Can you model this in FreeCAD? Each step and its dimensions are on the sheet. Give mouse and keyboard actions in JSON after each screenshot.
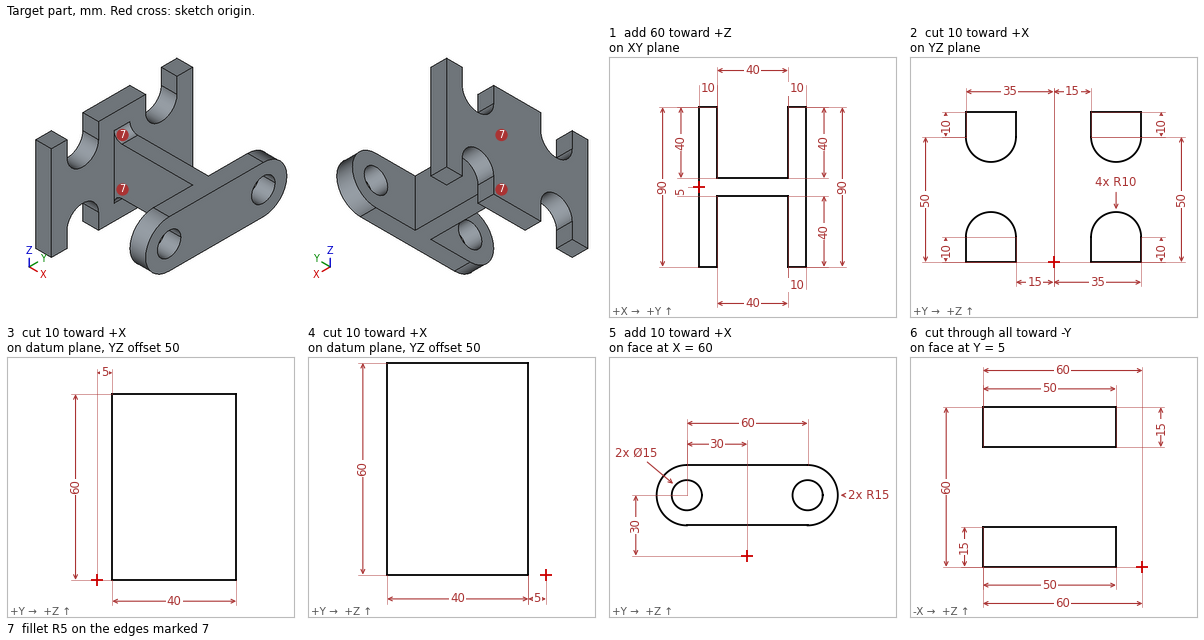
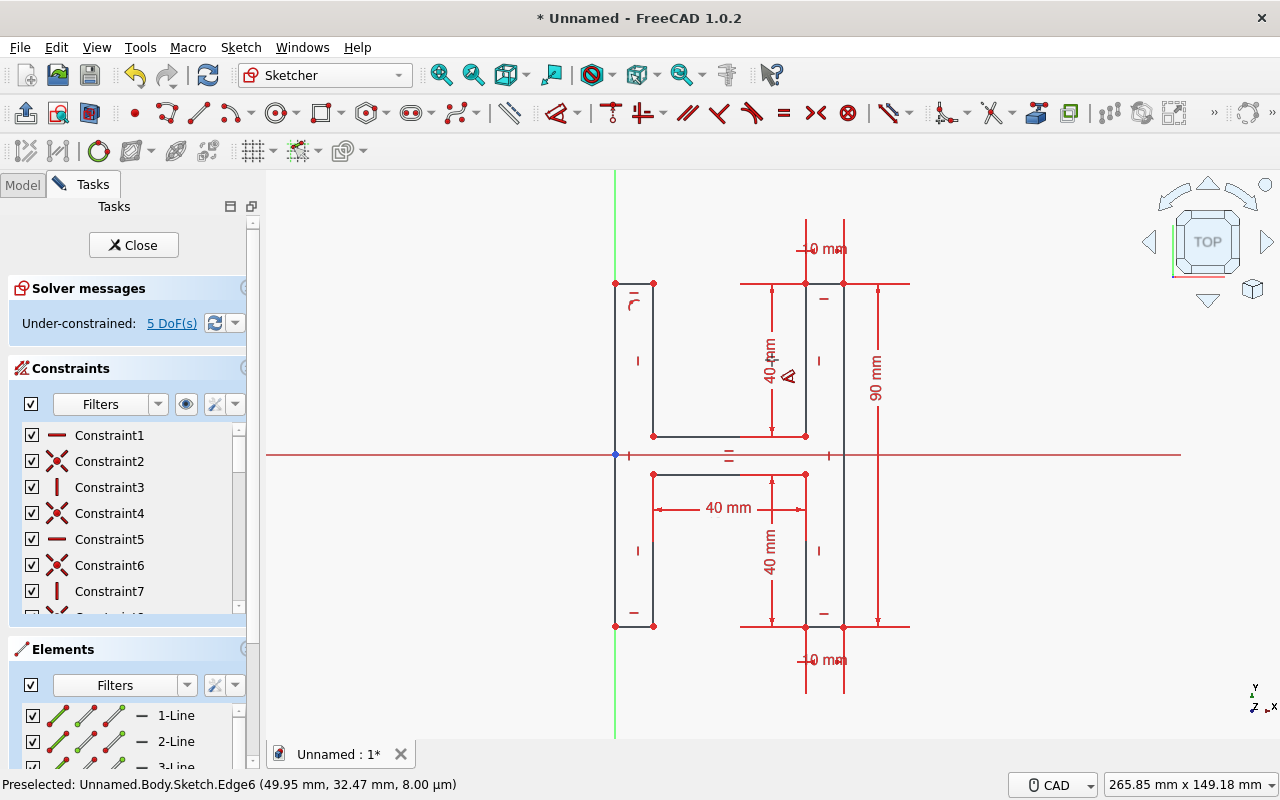
{"action": "left_click", "coordinate": [760, 437]}
{"action": "left_click", "coordinate": [729, 403]}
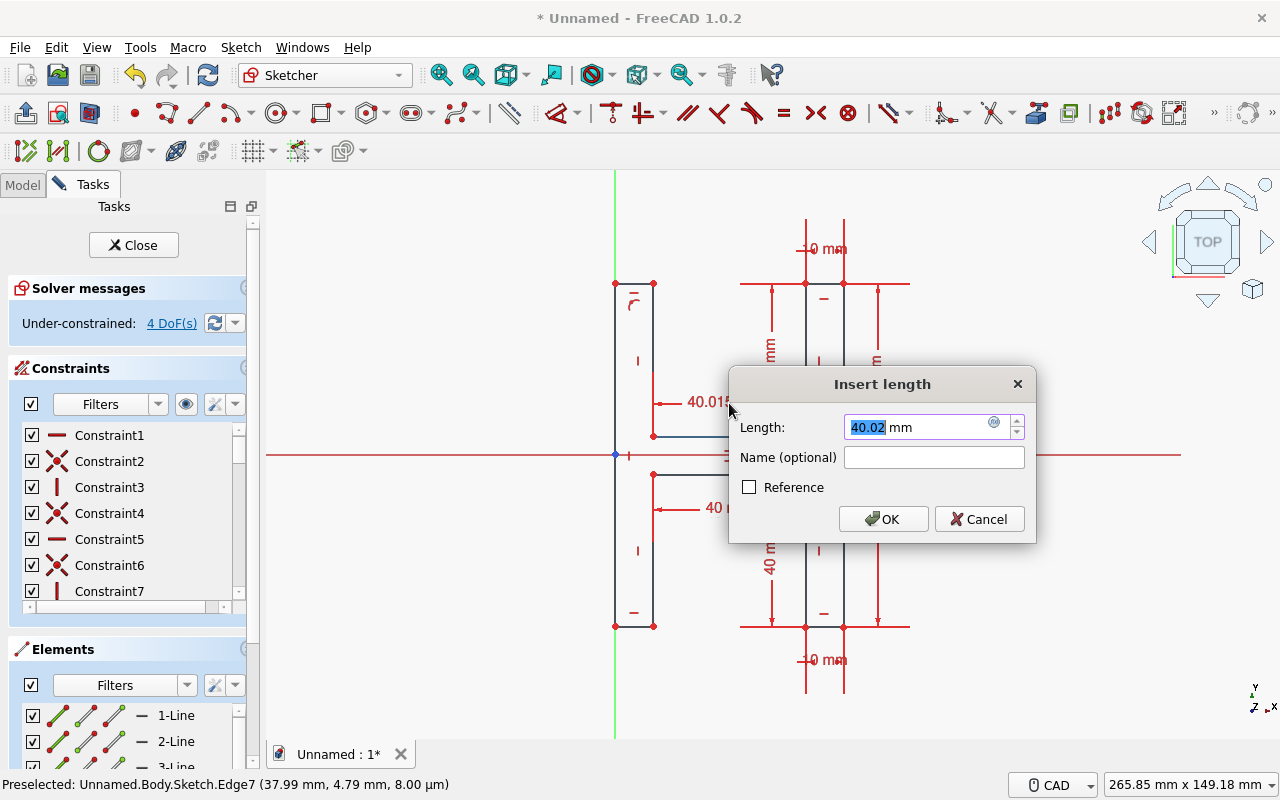
{"action": "type", "text": "40"}
{"action": "key", "text": "Return"}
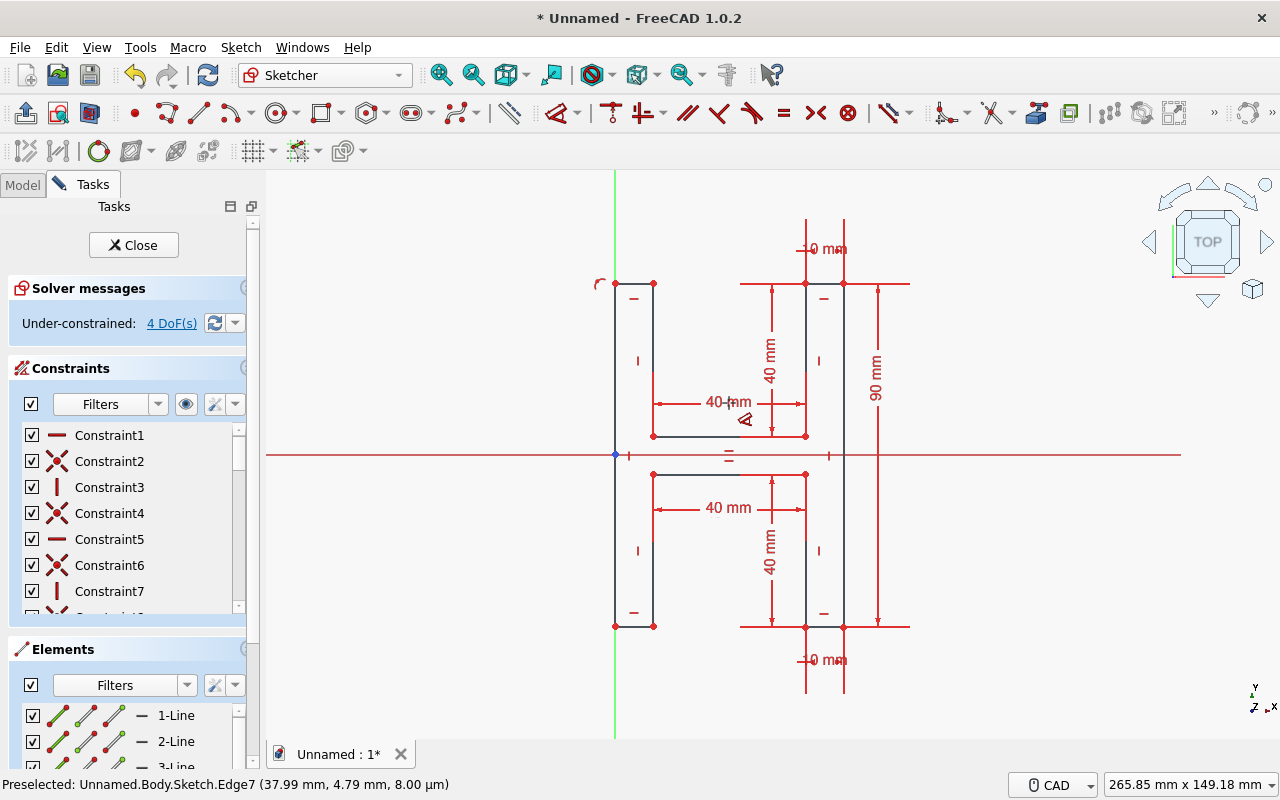
{"action": "left_click", "coordinate": [653, 391]}
{"action": "left_click", "coordinate": [687, 360]}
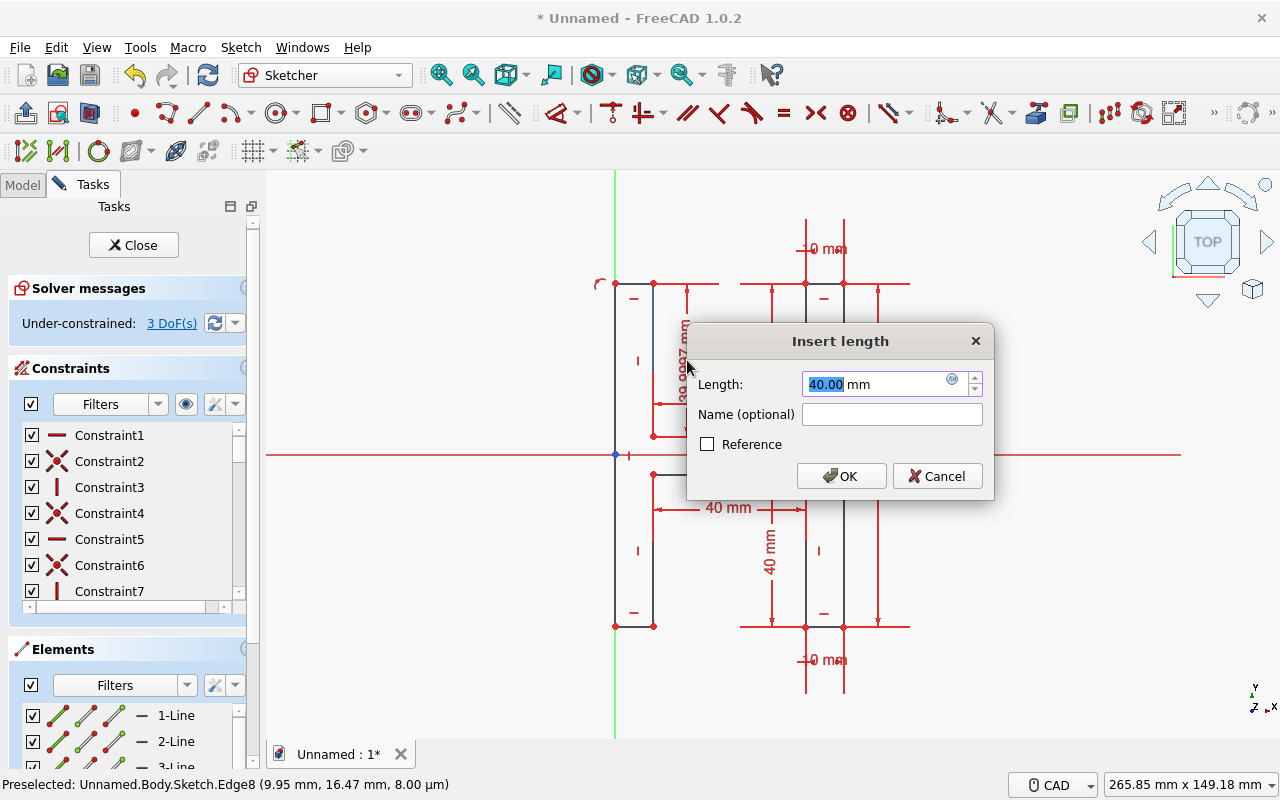
{"action": "type", "text": "40"}
{"action": "key", "text": "Return"}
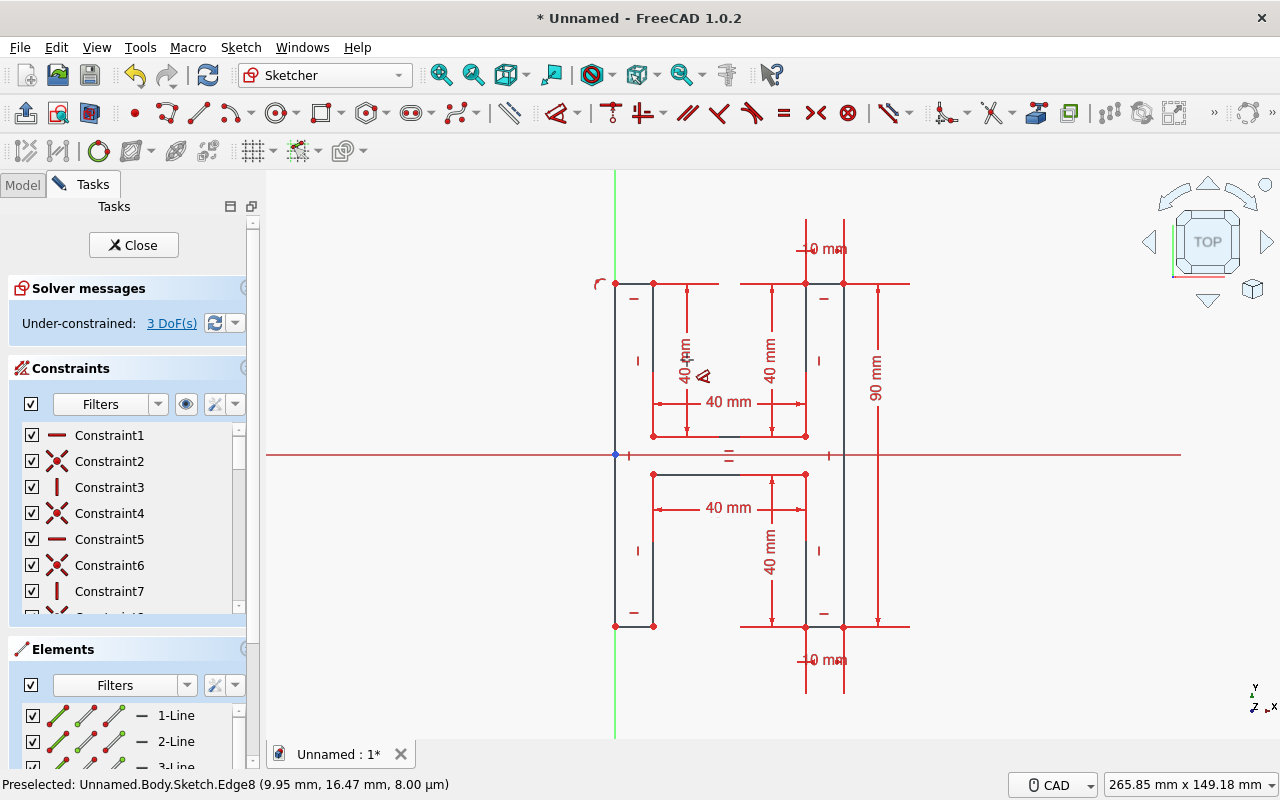
{"action": "left_click", "coordinate": [642, 284]}
{"action": "left_click", "coordinate": [634, 250]}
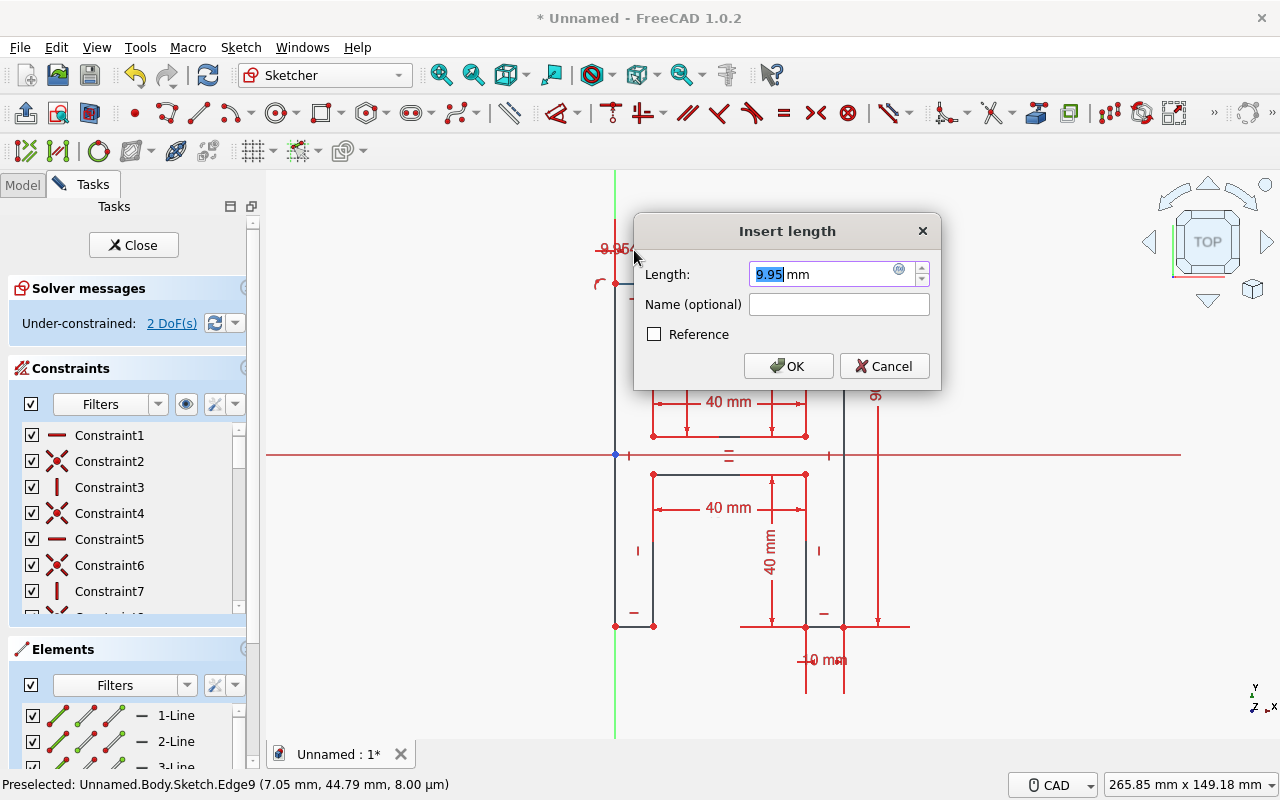
{"action": "type", "text": "10"}
{"action": "key", "text": "Return"}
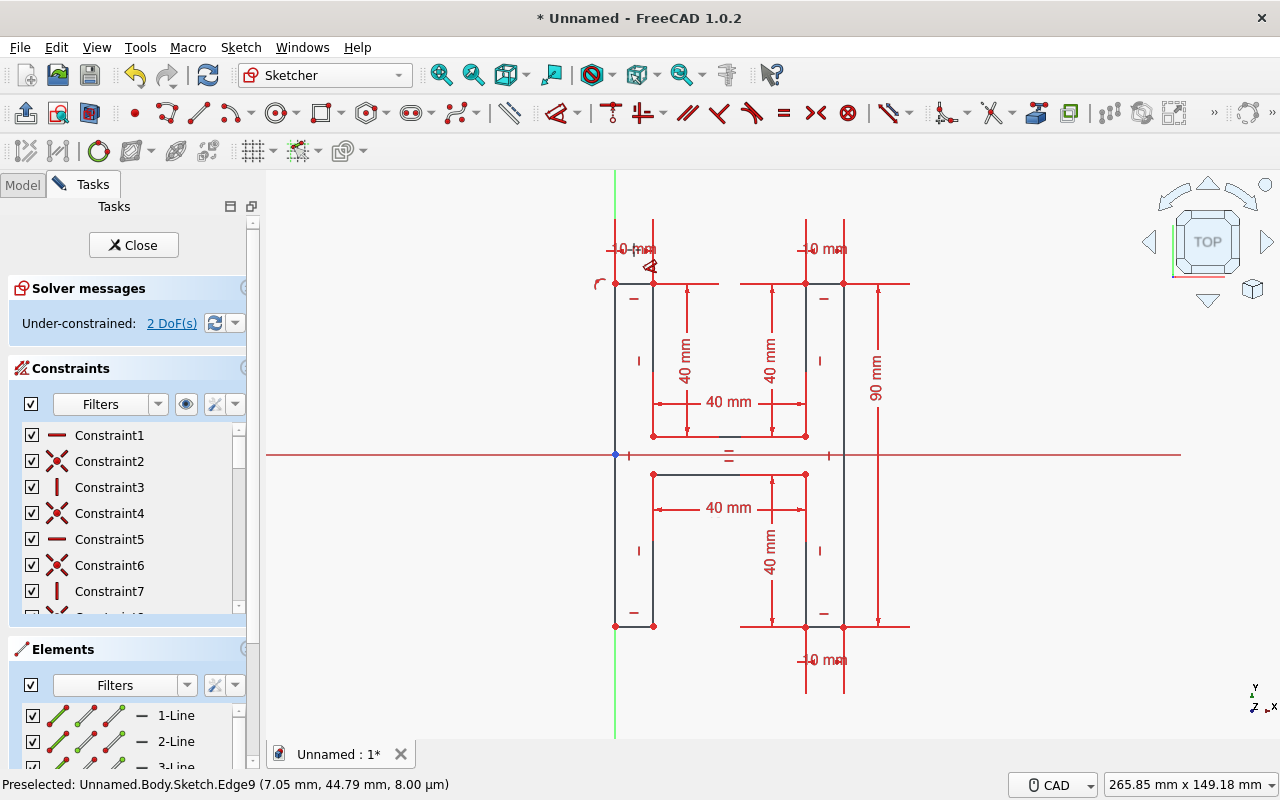
{"action": "left_click", "coordinate": [615, 387]}
{"action": "left_click", "coordinate": [581, 377]}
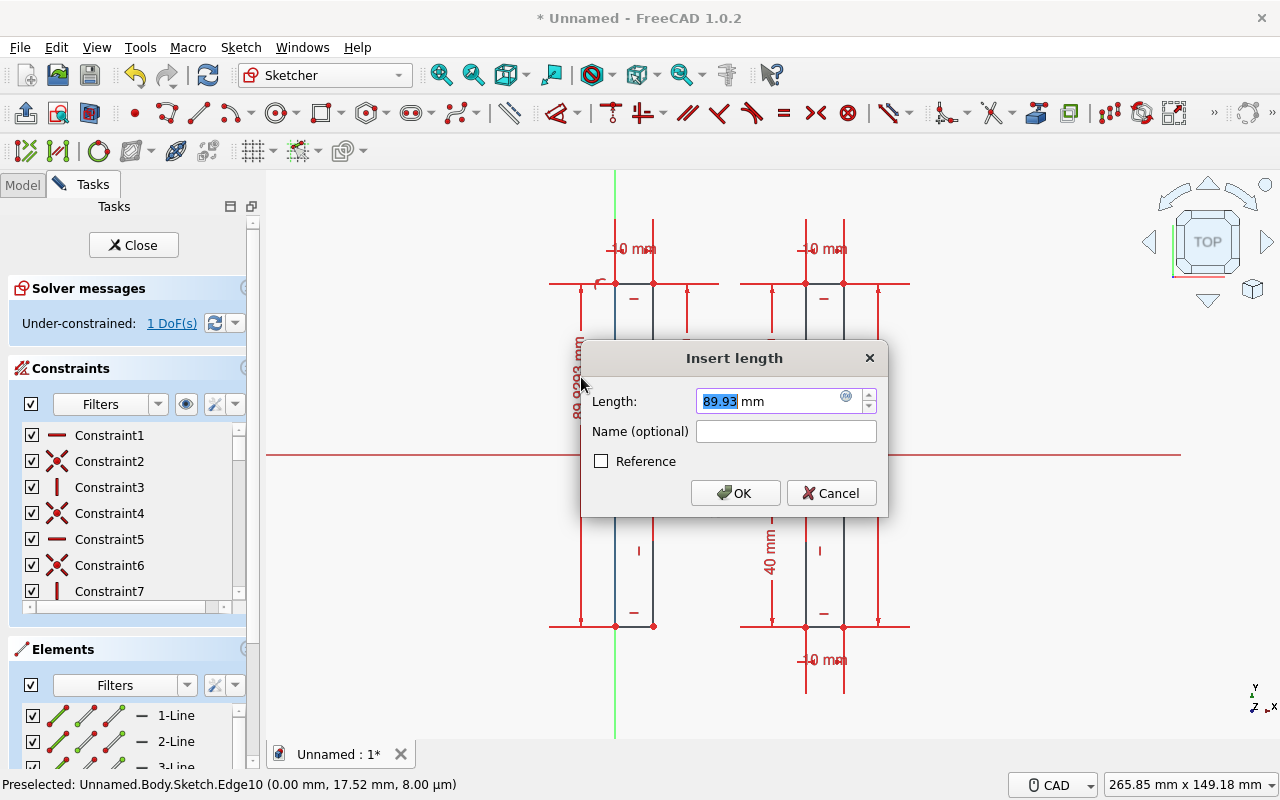
{"action": "type", "text": "90"}
{"action": "key", "text": "Return"}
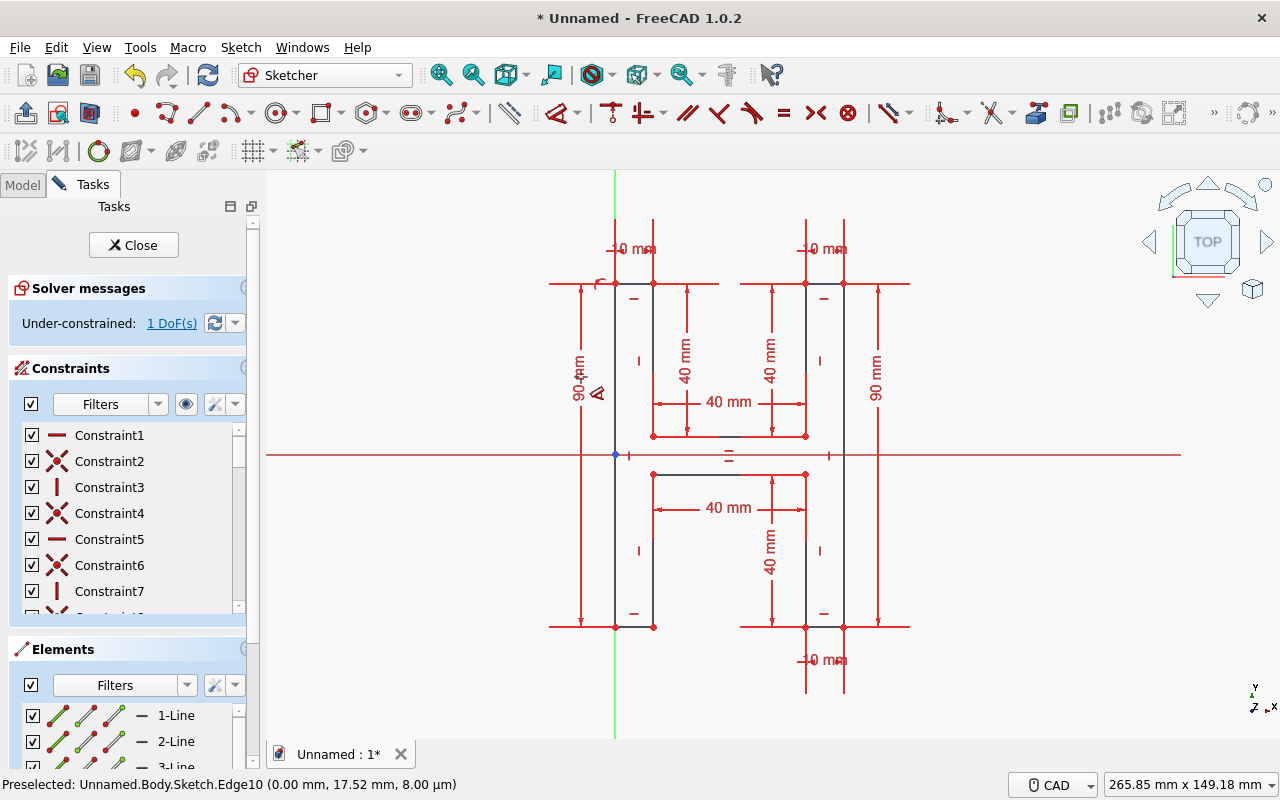
{"action": "scroll", "coordinate": [653, 475], "scroll_direction": "up", "scroll_amount": 4}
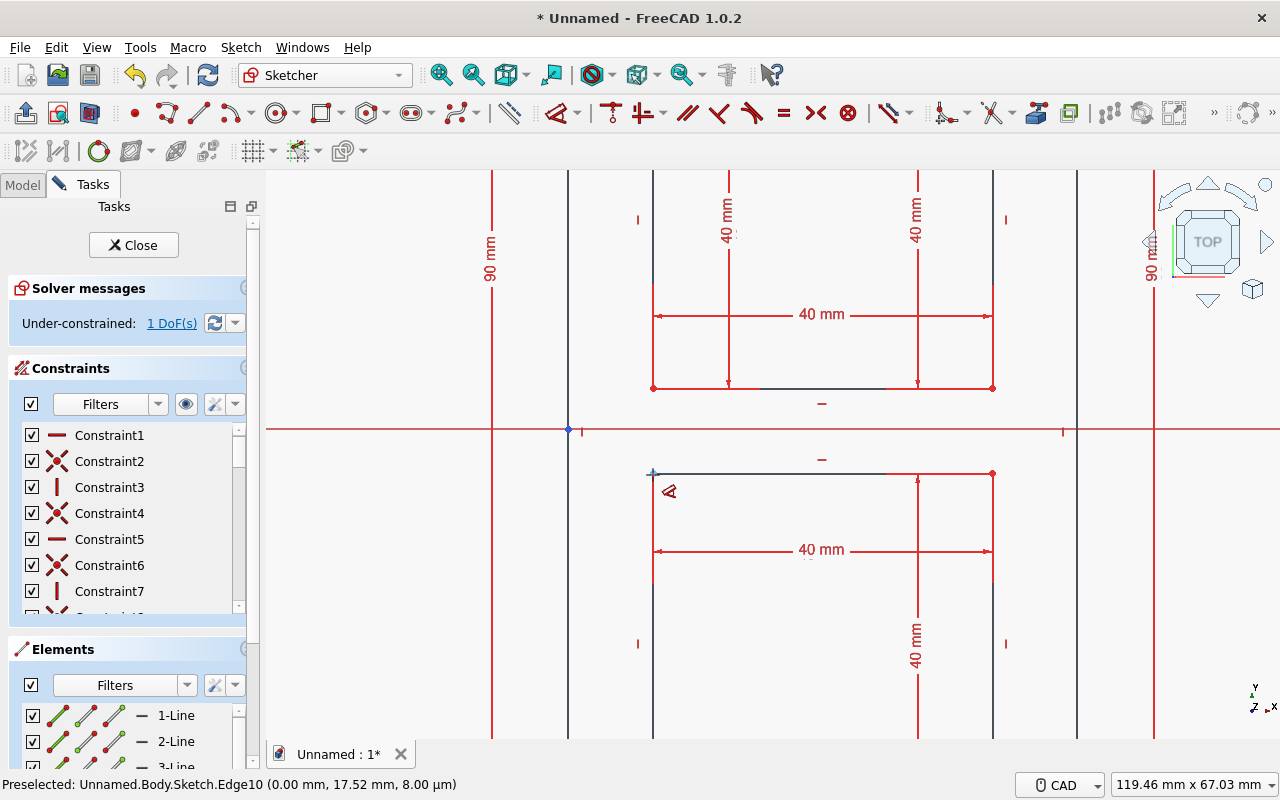
{"action": "left_click", "coordinate": [653, 474]}
{"action": "left_click", "coordinate": [534, 452]}